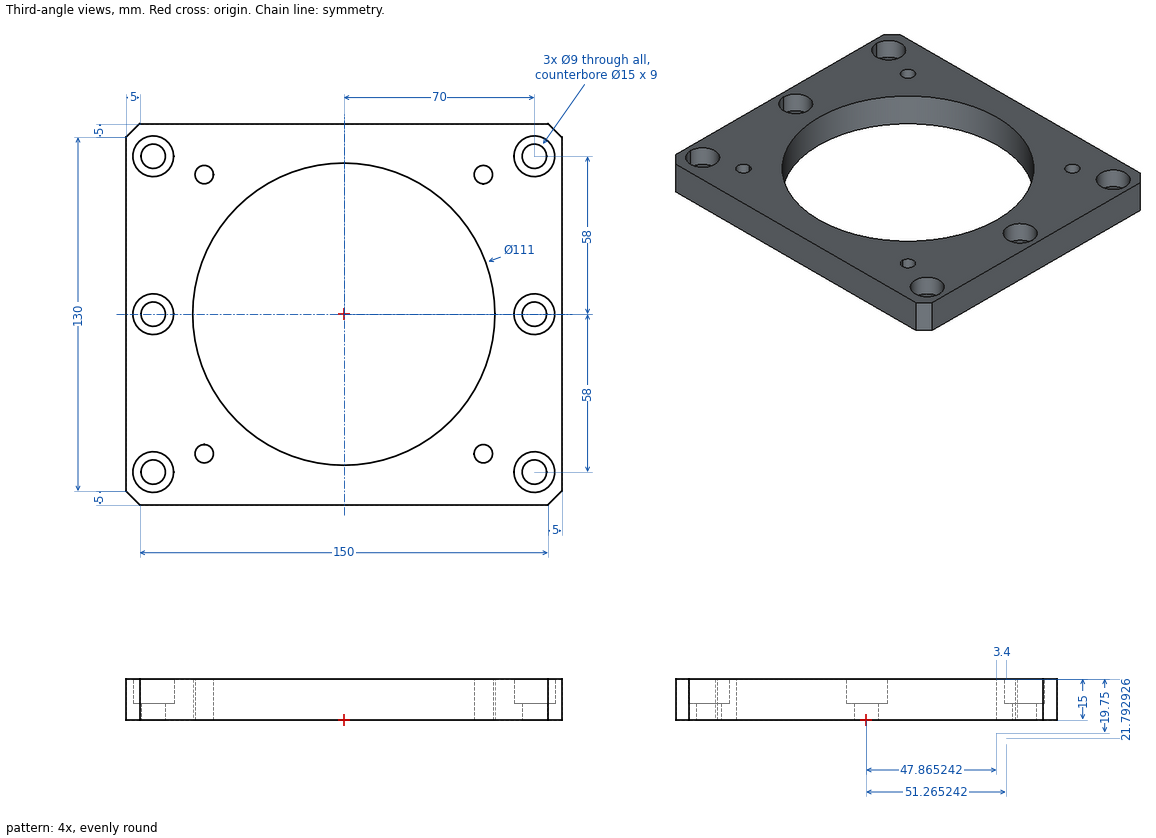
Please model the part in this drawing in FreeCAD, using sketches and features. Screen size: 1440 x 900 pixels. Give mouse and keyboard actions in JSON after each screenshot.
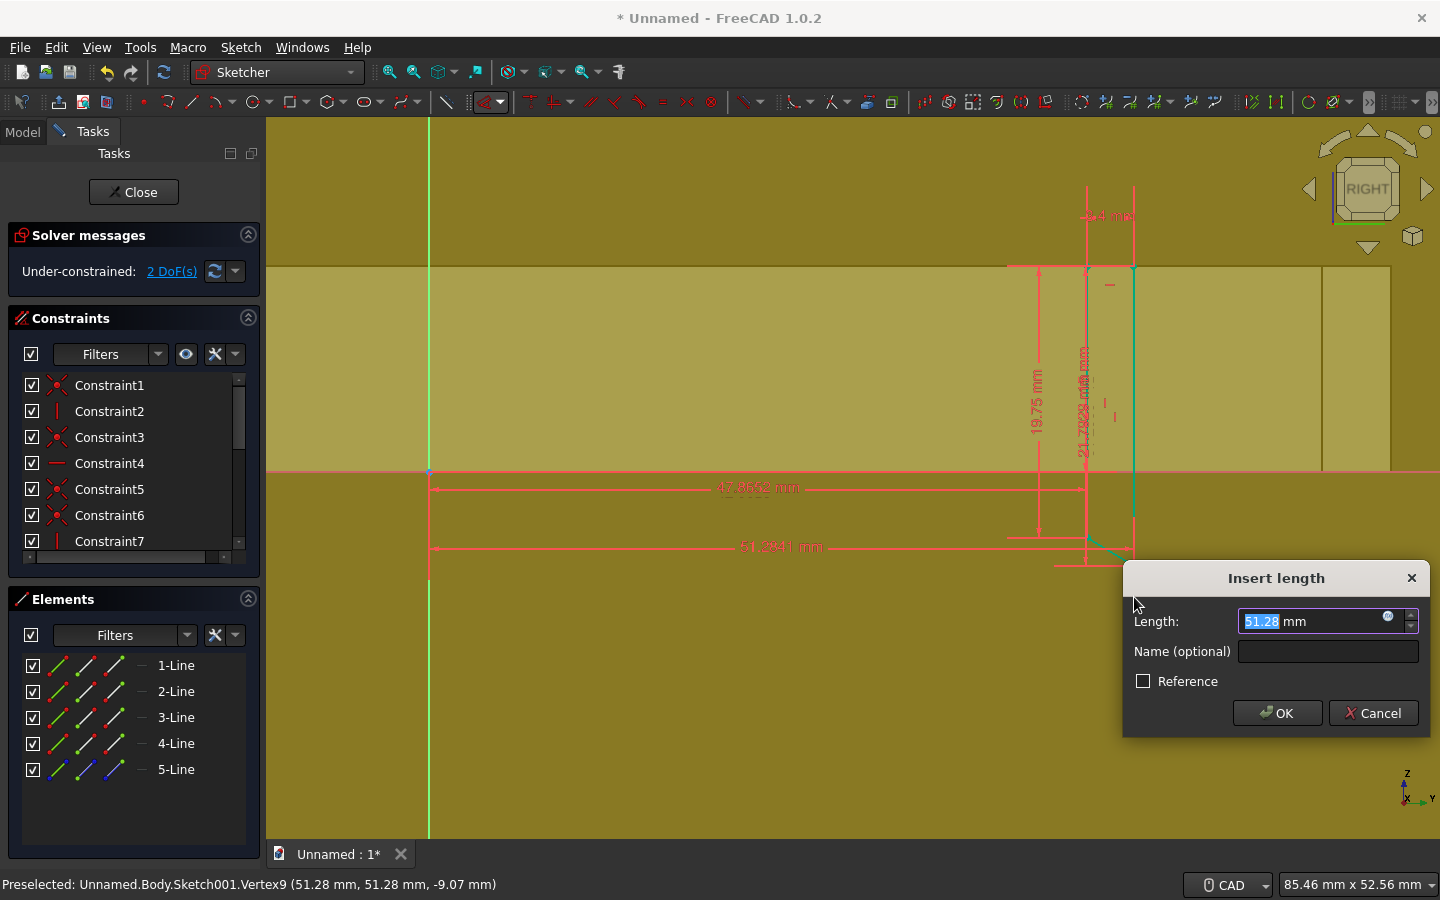
{"action": "type", "text": "51.265242"}
{"action": "key", "text": "Return"}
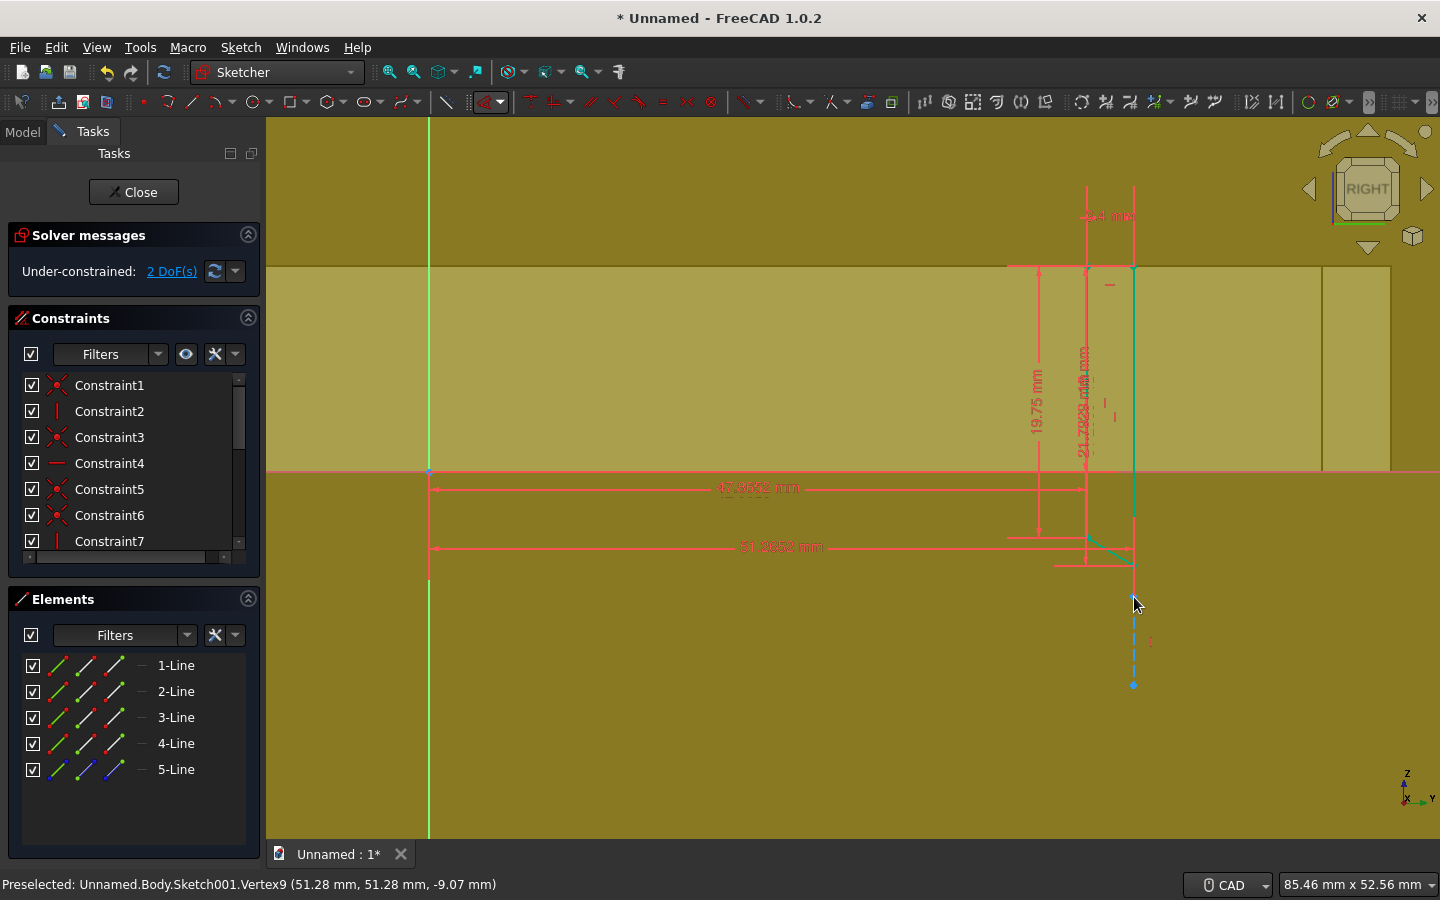
{"action": "left_click", "coordinate": [134, 192]}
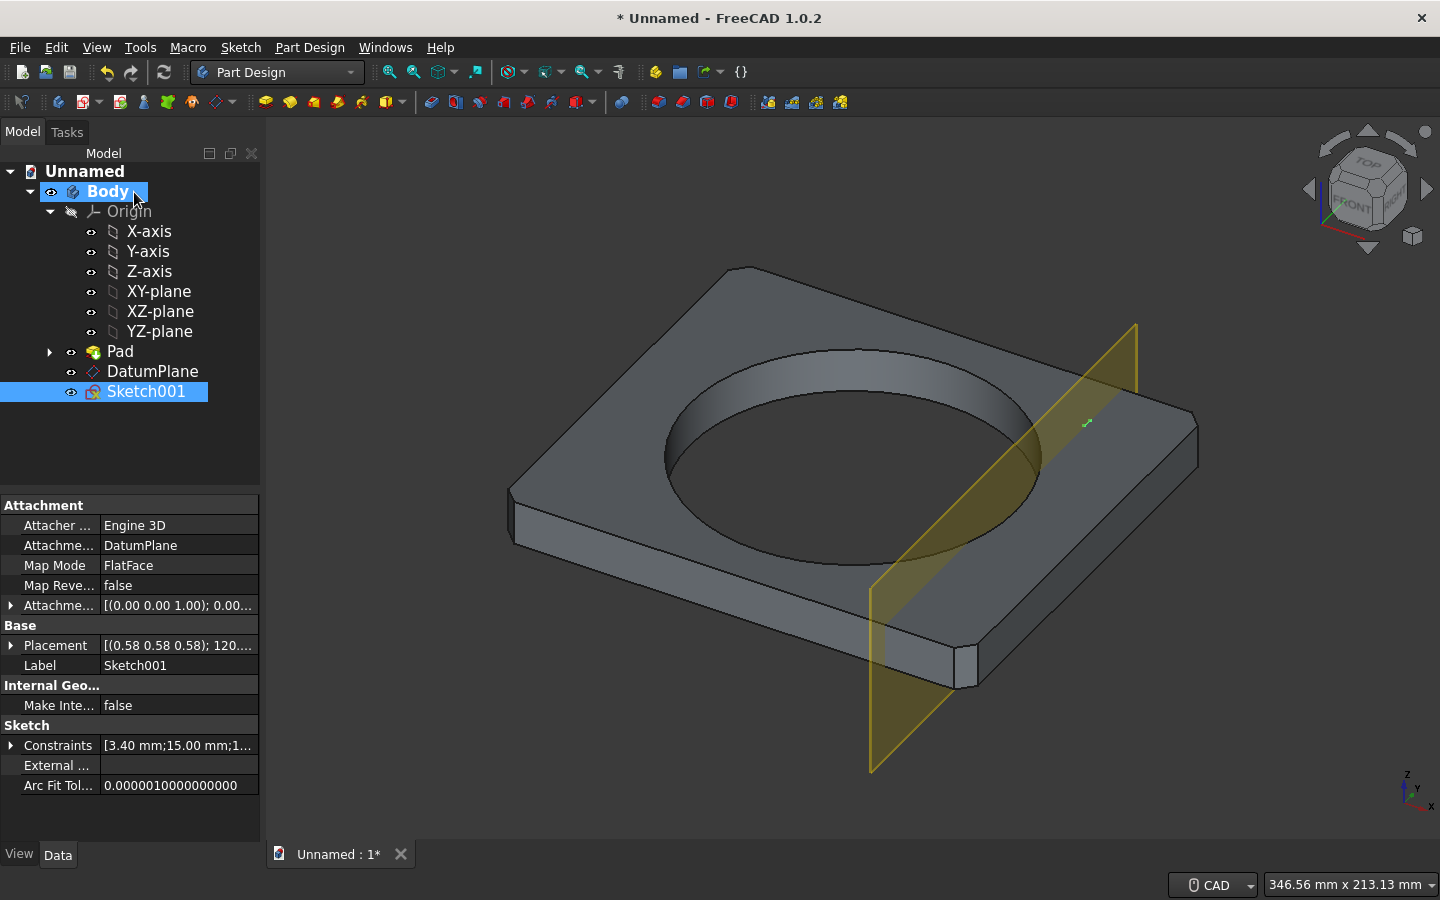
{"action": "left_click", "coordinate": [480, 102]}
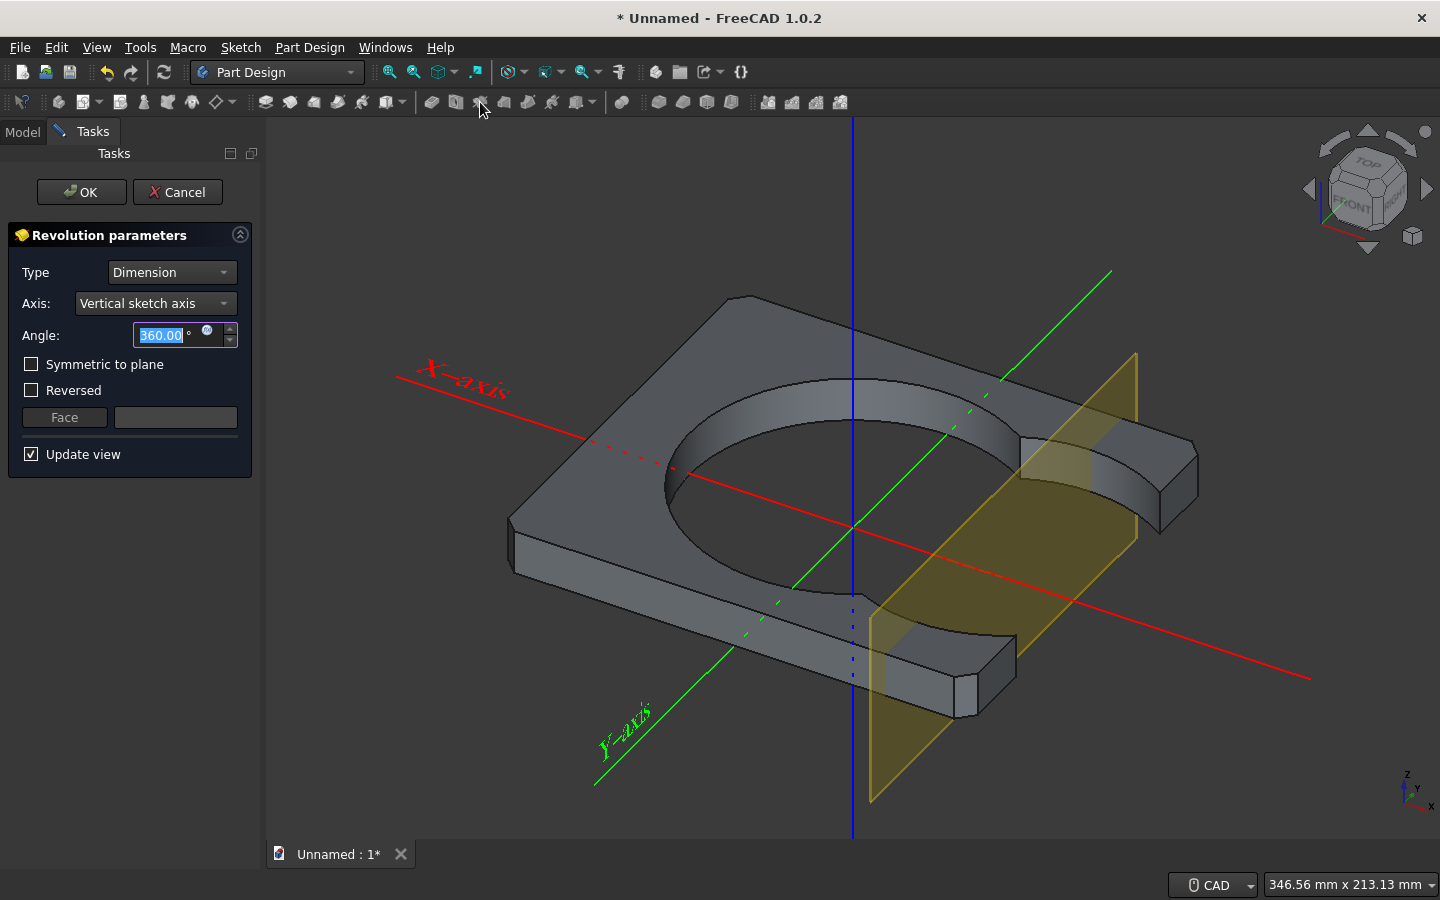
{"action": "left_click", "coordinate": [156, 304]}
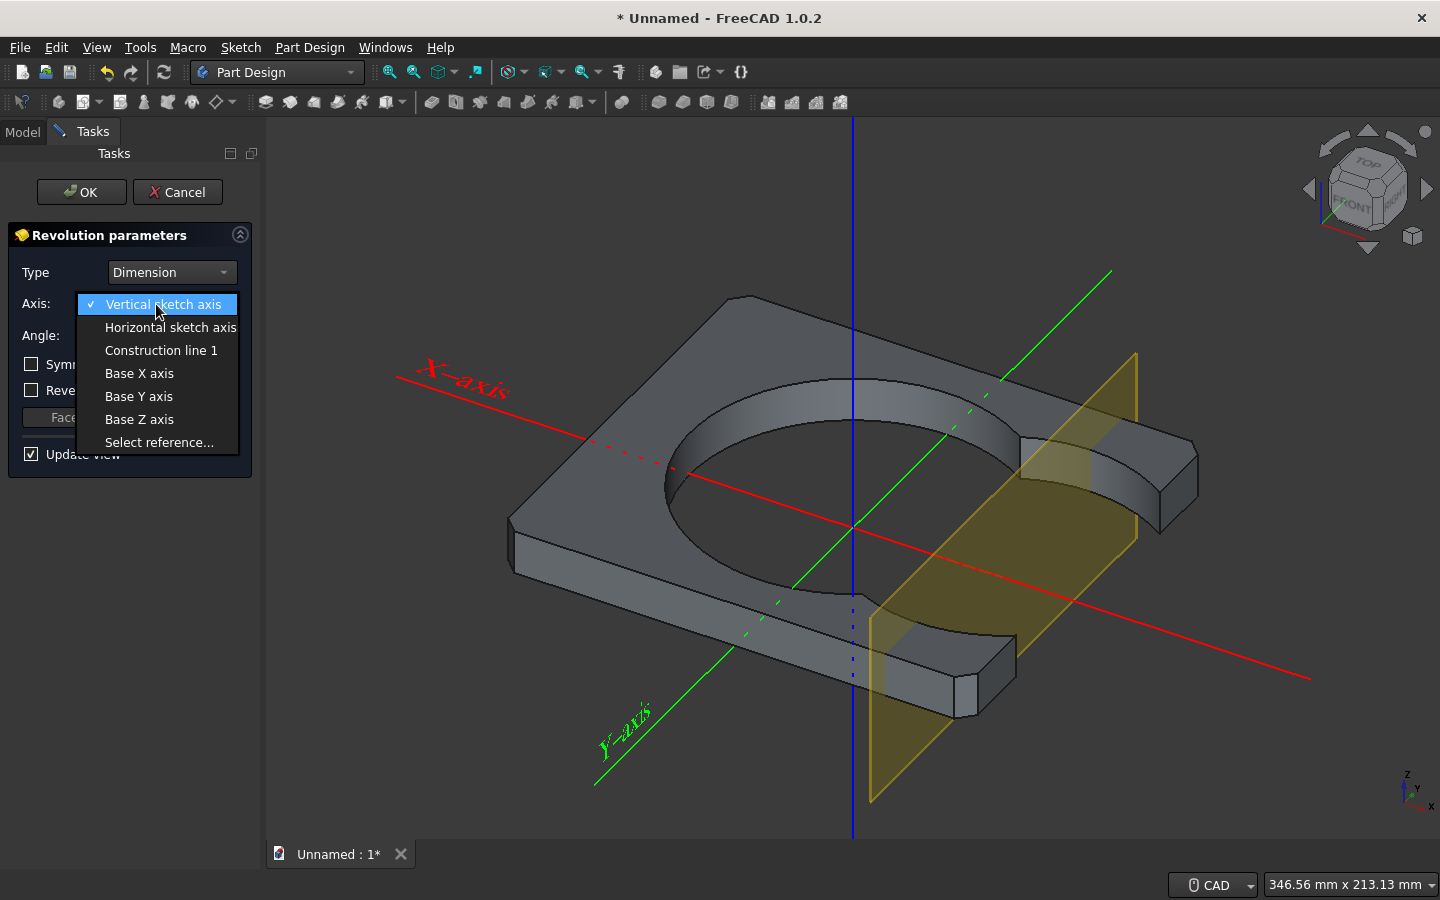
{"action": "left_click", "coordinate": [156, 350]}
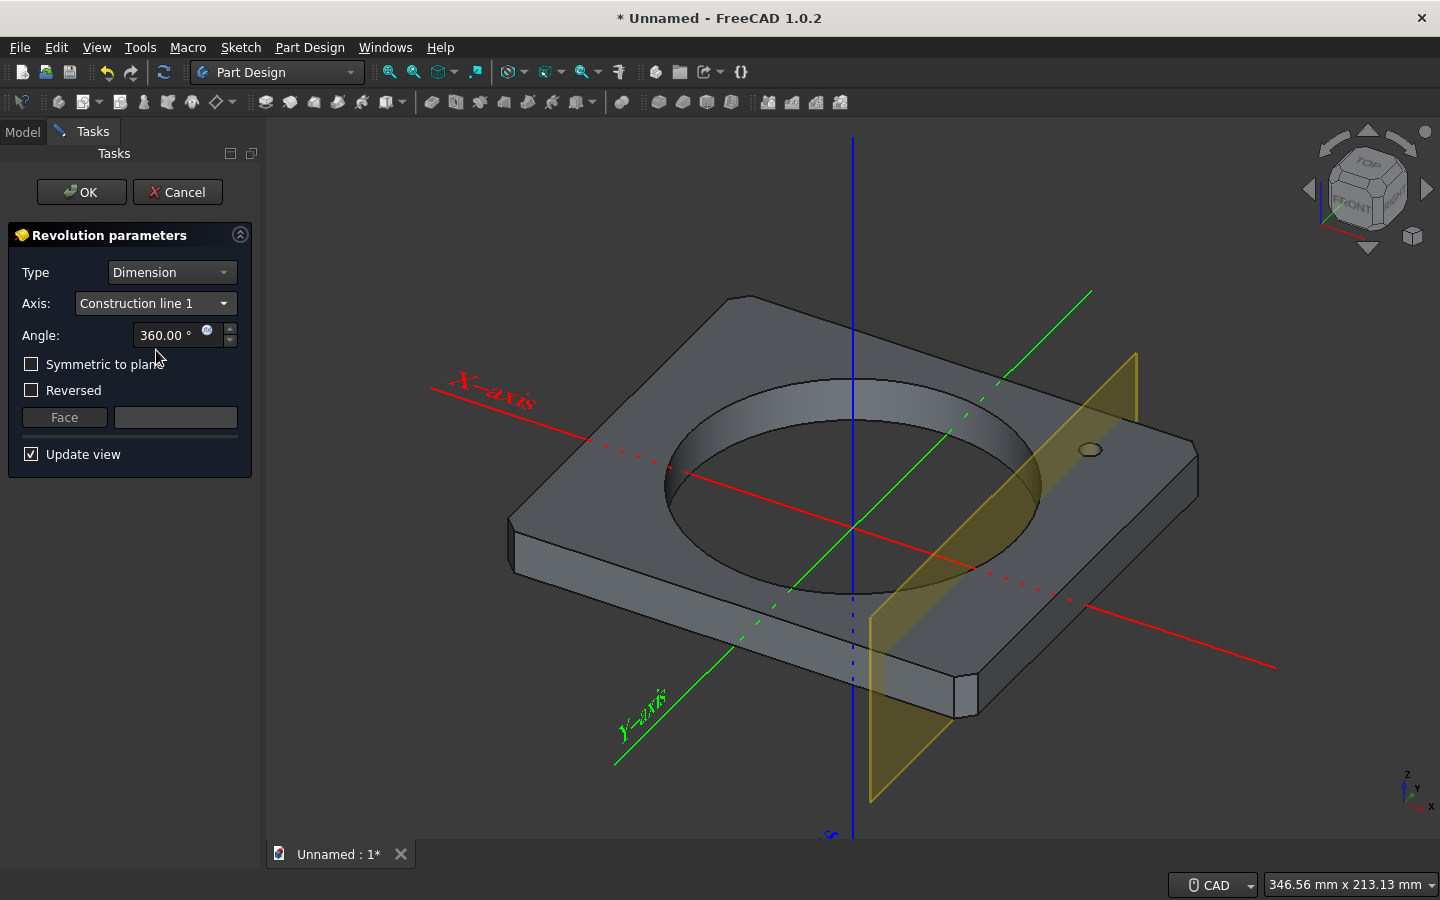
{"action": "left_click", "coordinate": [82, 192]}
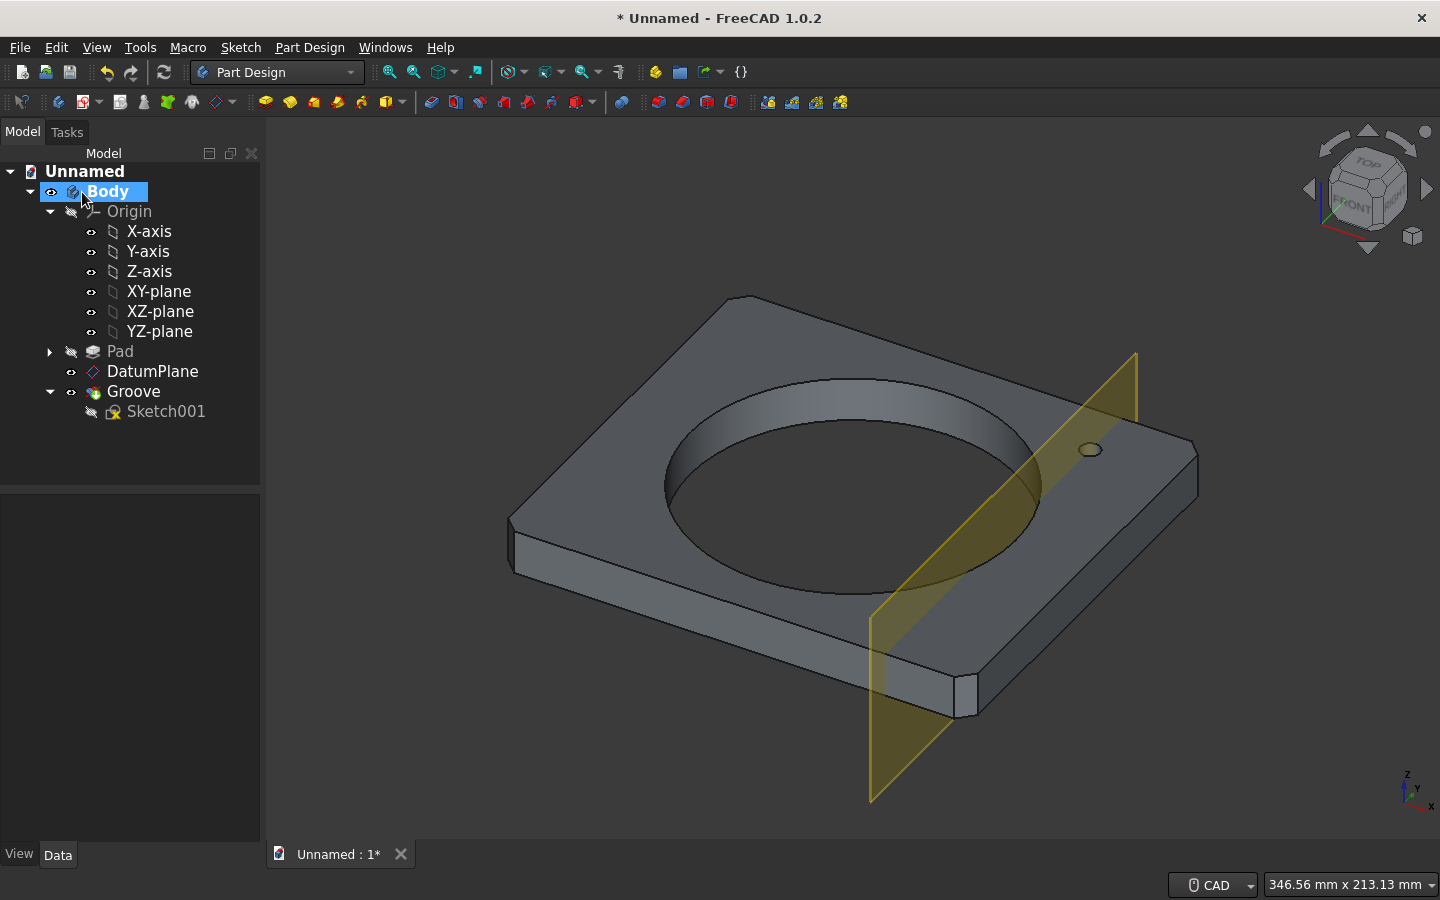
{"action": "left_click", "coordinate": [116, 372]}
{"action": "key", "text": "space"}